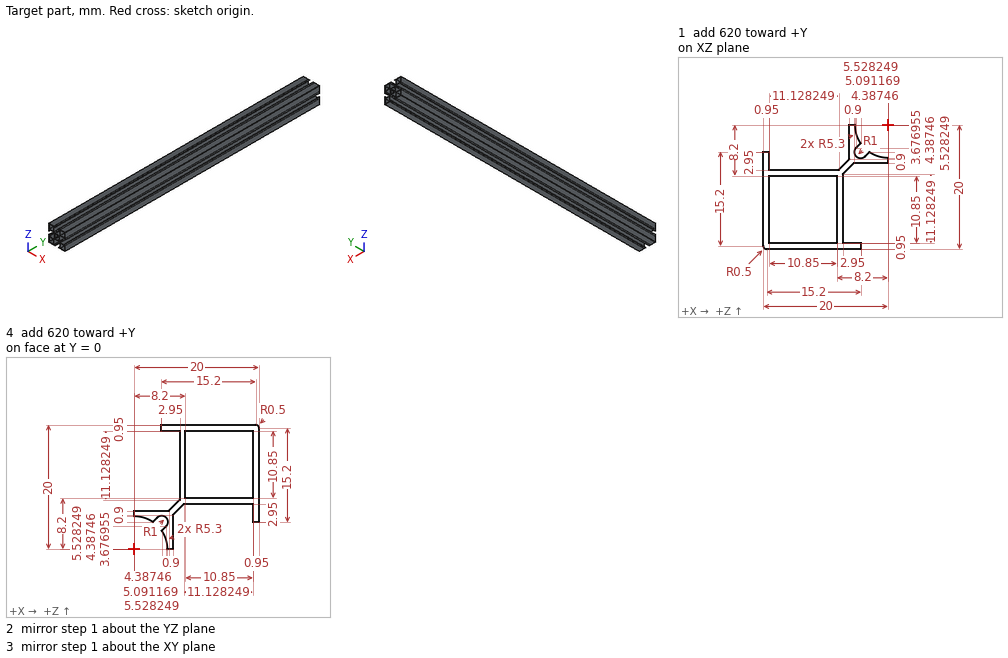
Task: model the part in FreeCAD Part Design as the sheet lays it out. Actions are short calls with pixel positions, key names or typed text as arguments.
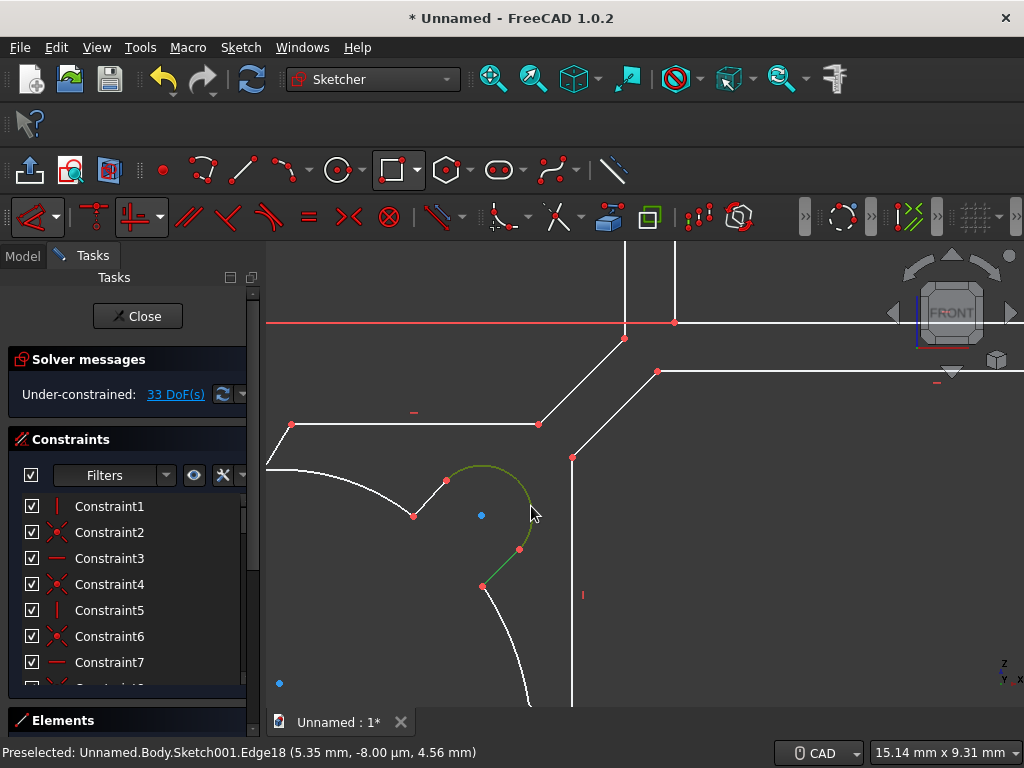
click(270, 218)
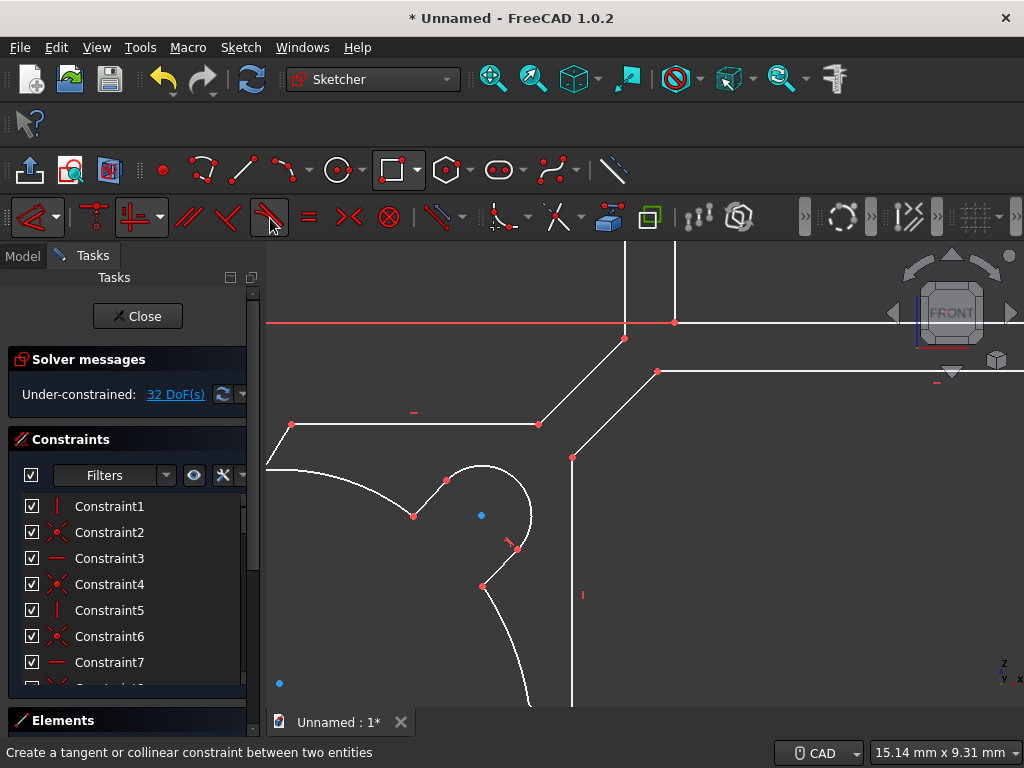
click(437, 491)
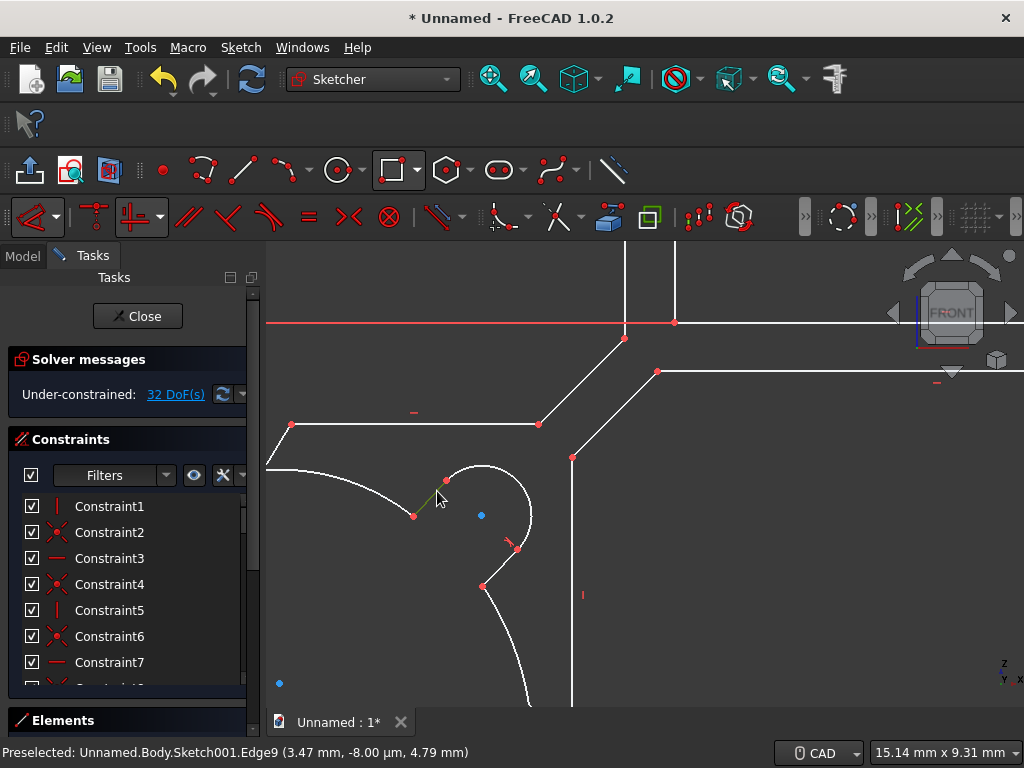
click(531, 507)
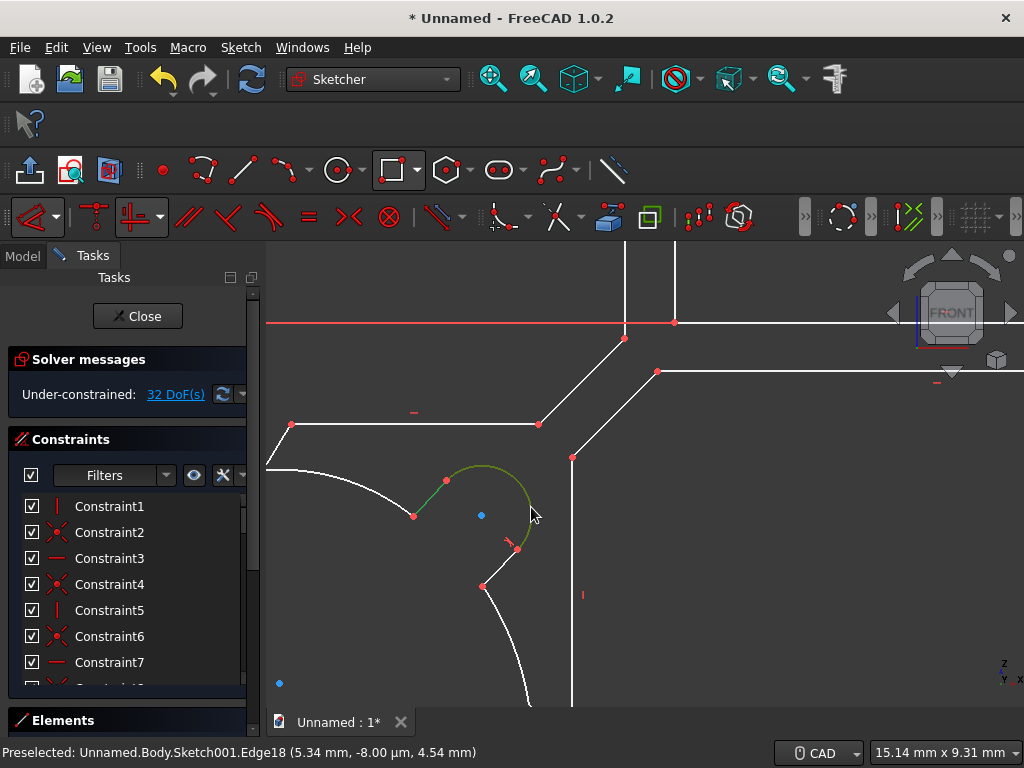
click(270, 218)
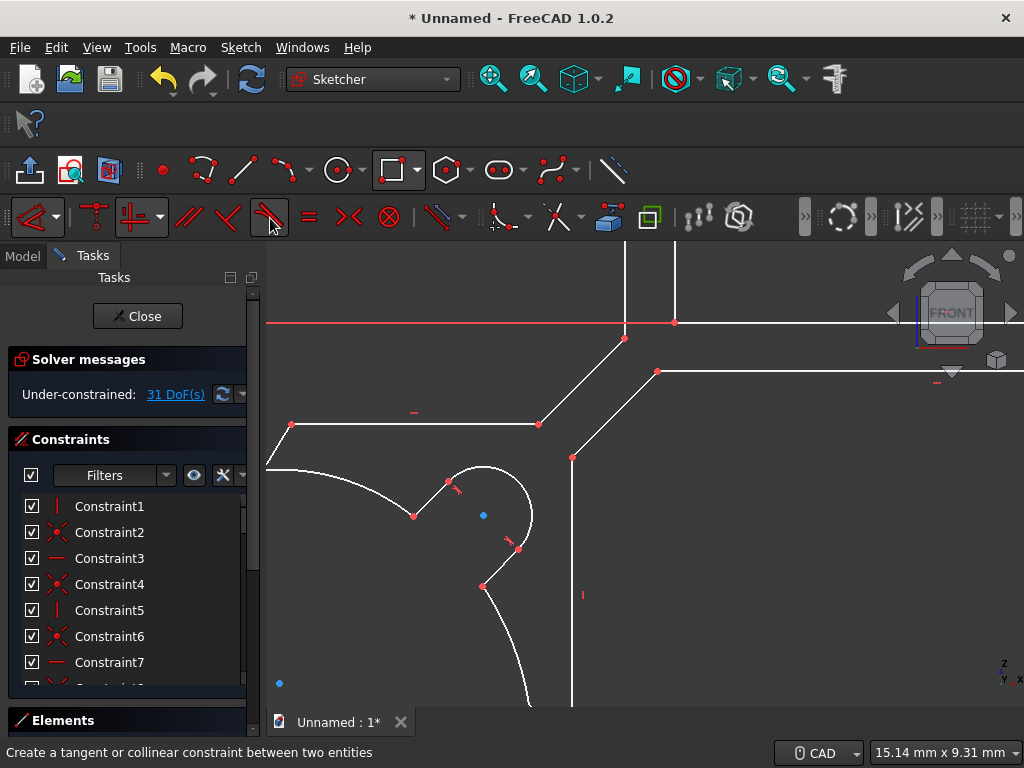
scroll(496, 579, down, 6)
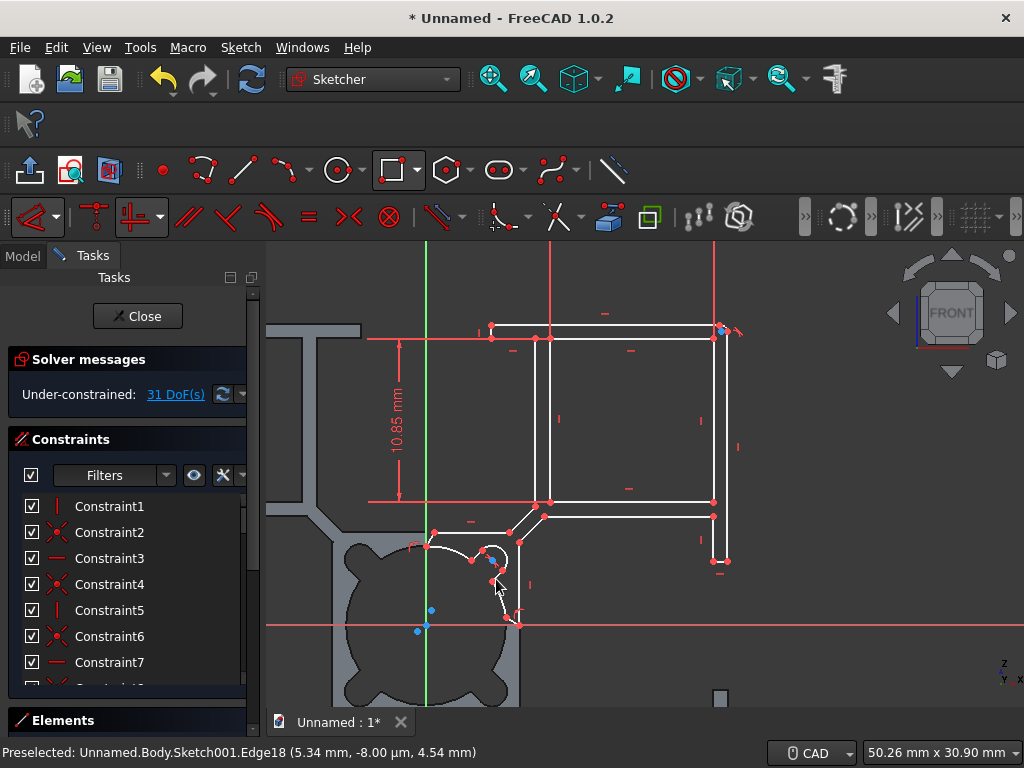
click(560, 325)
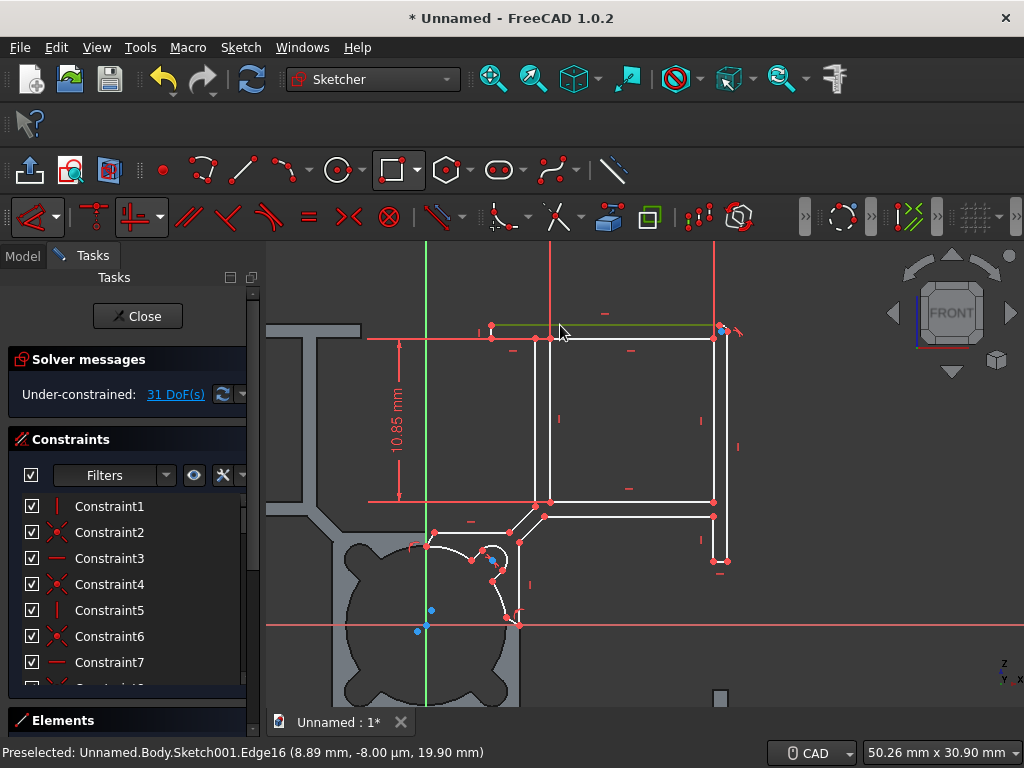
scroll(725, 327, up, 5)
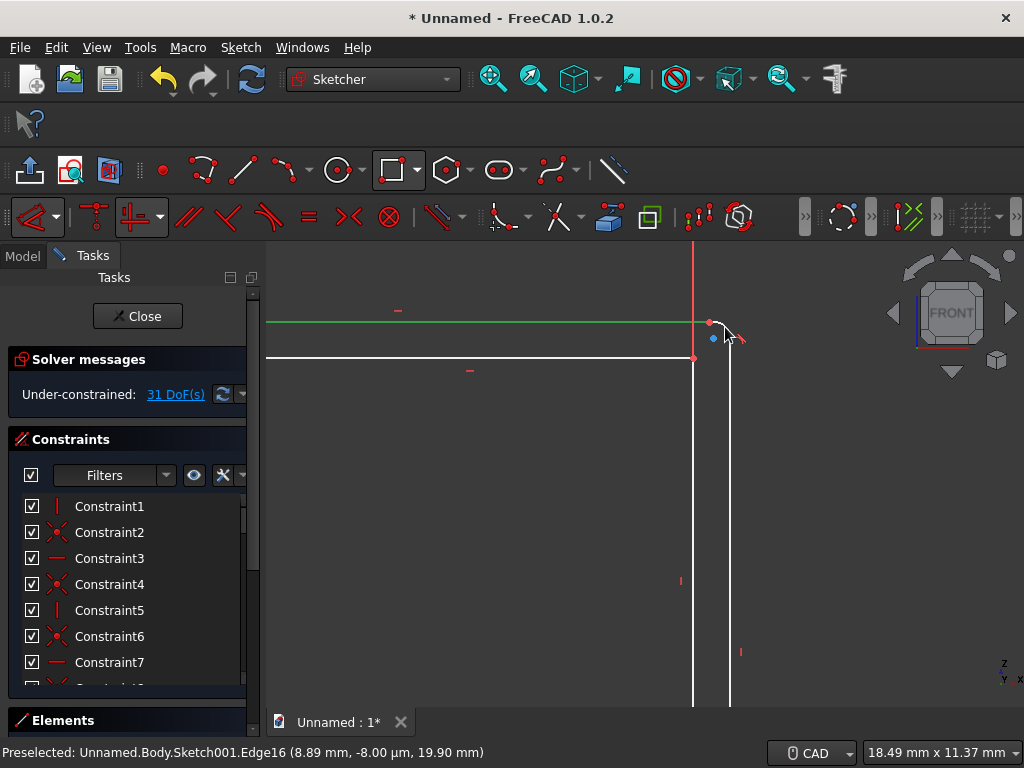
click(724, 325)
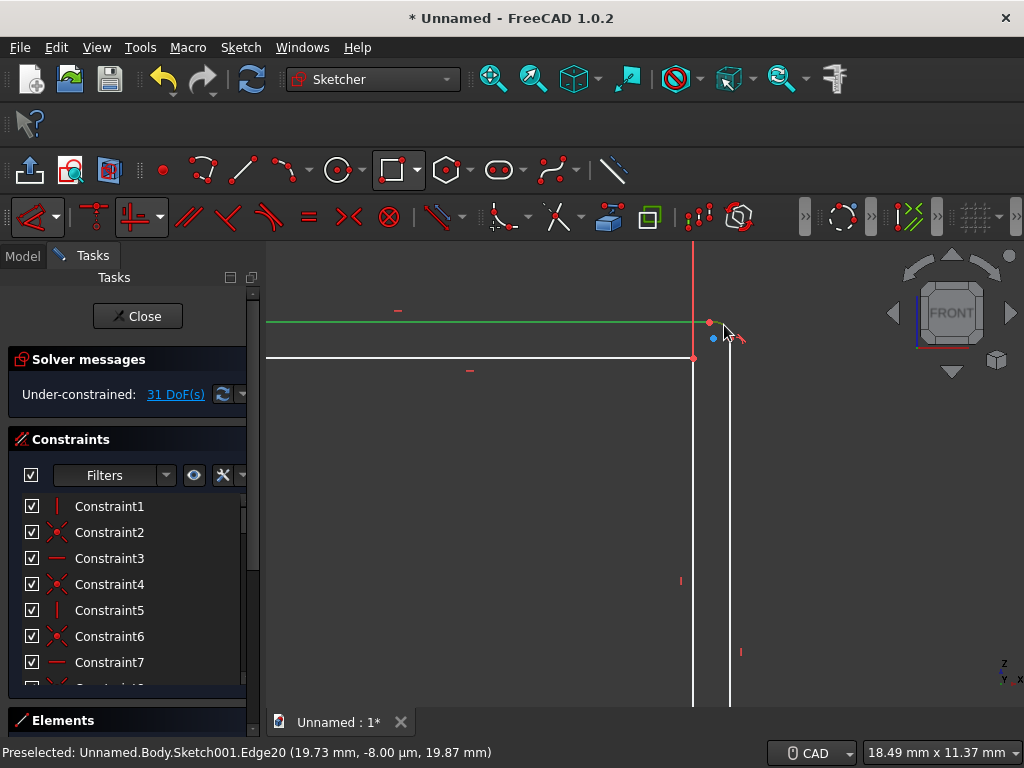
click(270, 218)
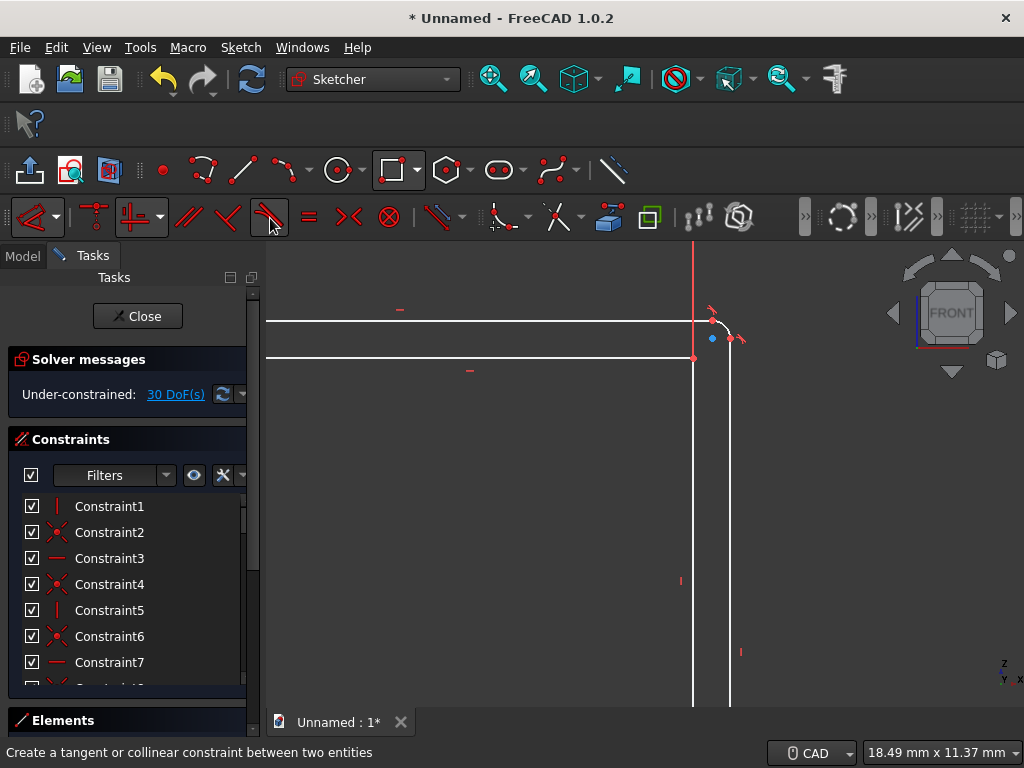
scroll(725, 326, down, 5)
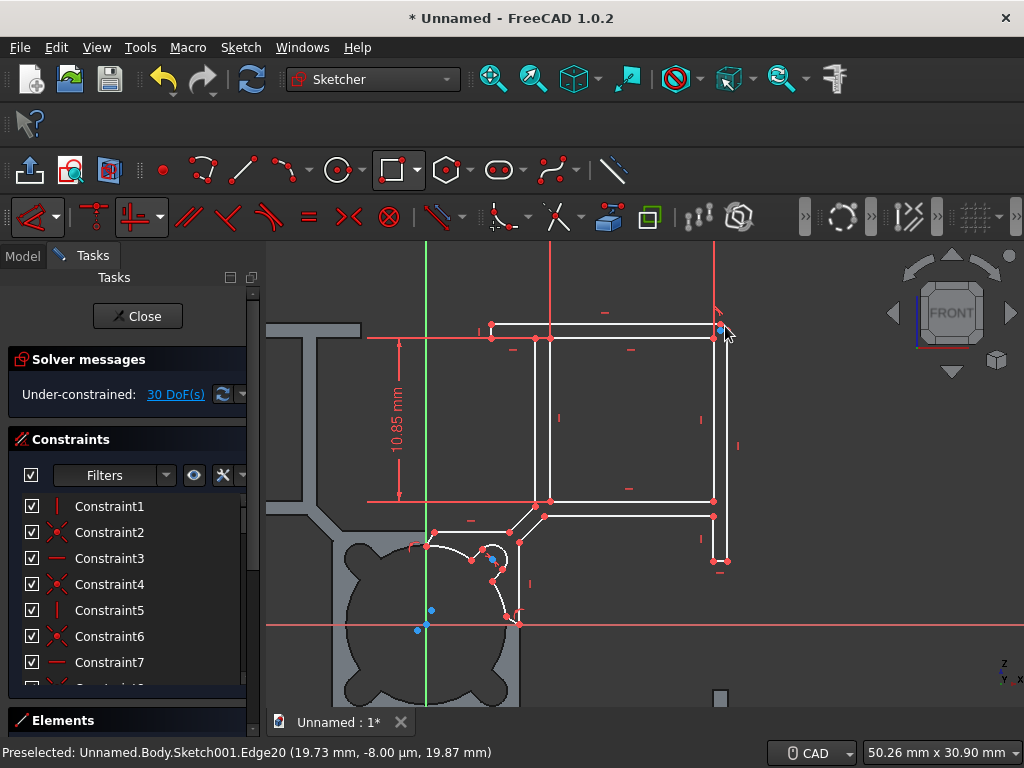
scroll(510, 619, up, 6)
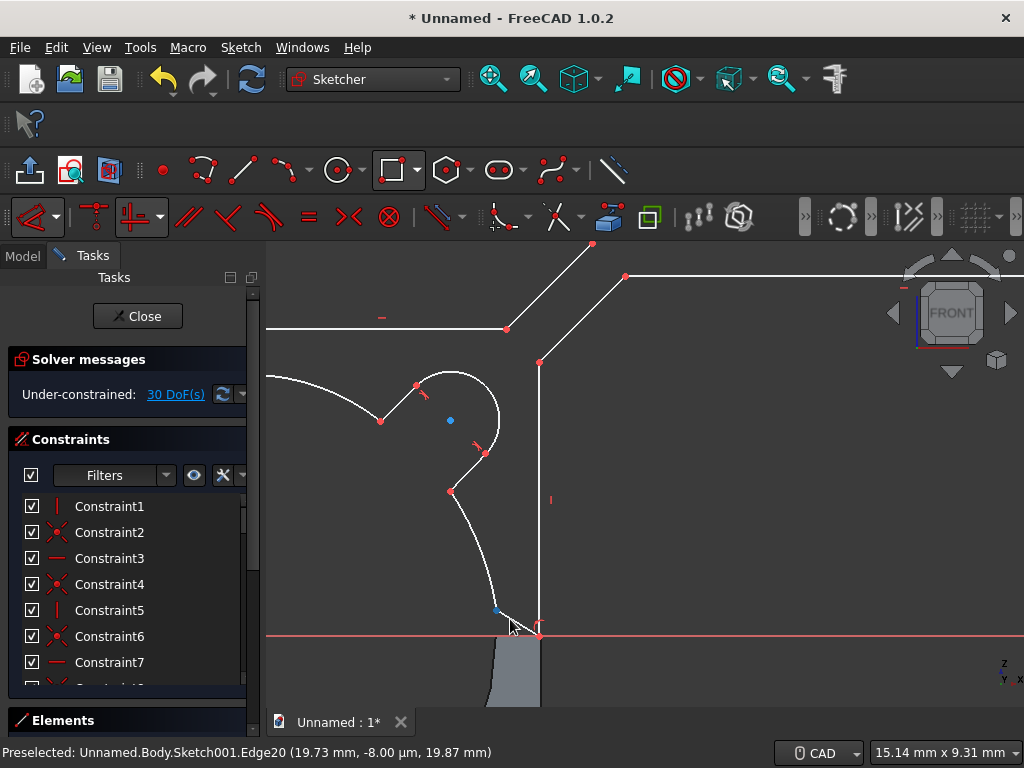
click(509, 618)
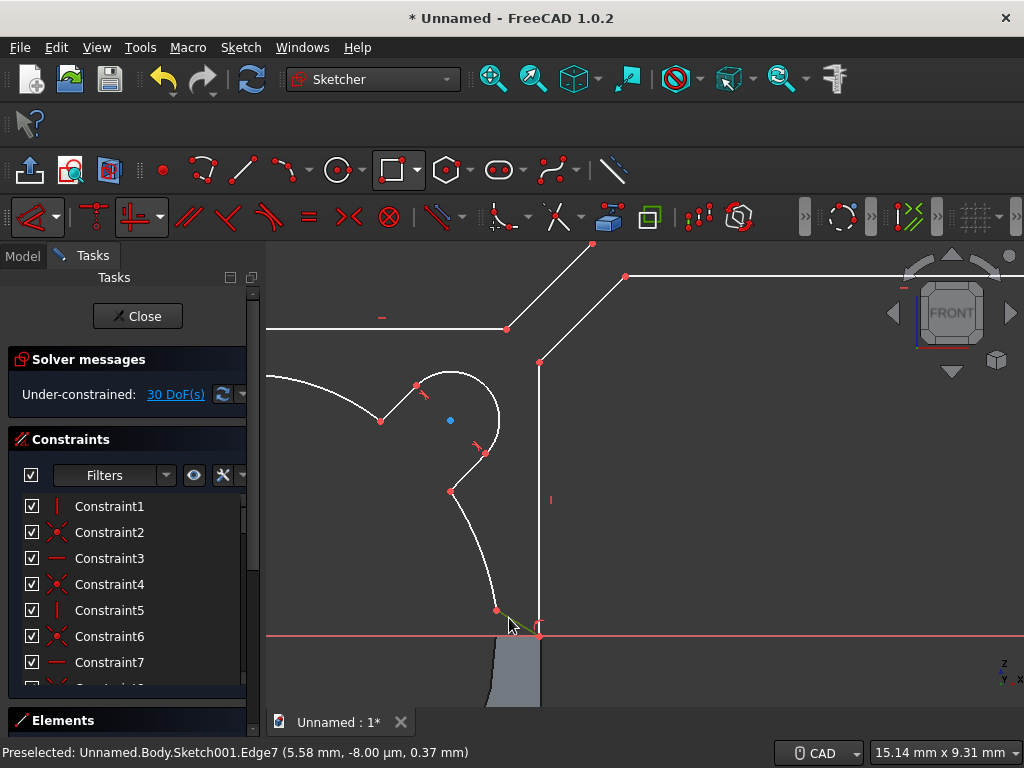
key(h)